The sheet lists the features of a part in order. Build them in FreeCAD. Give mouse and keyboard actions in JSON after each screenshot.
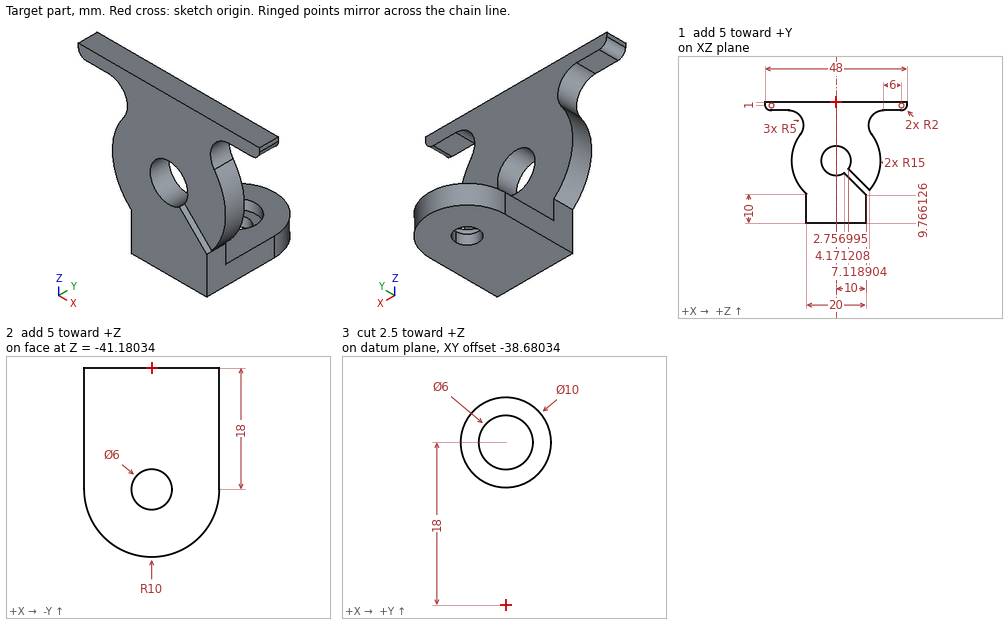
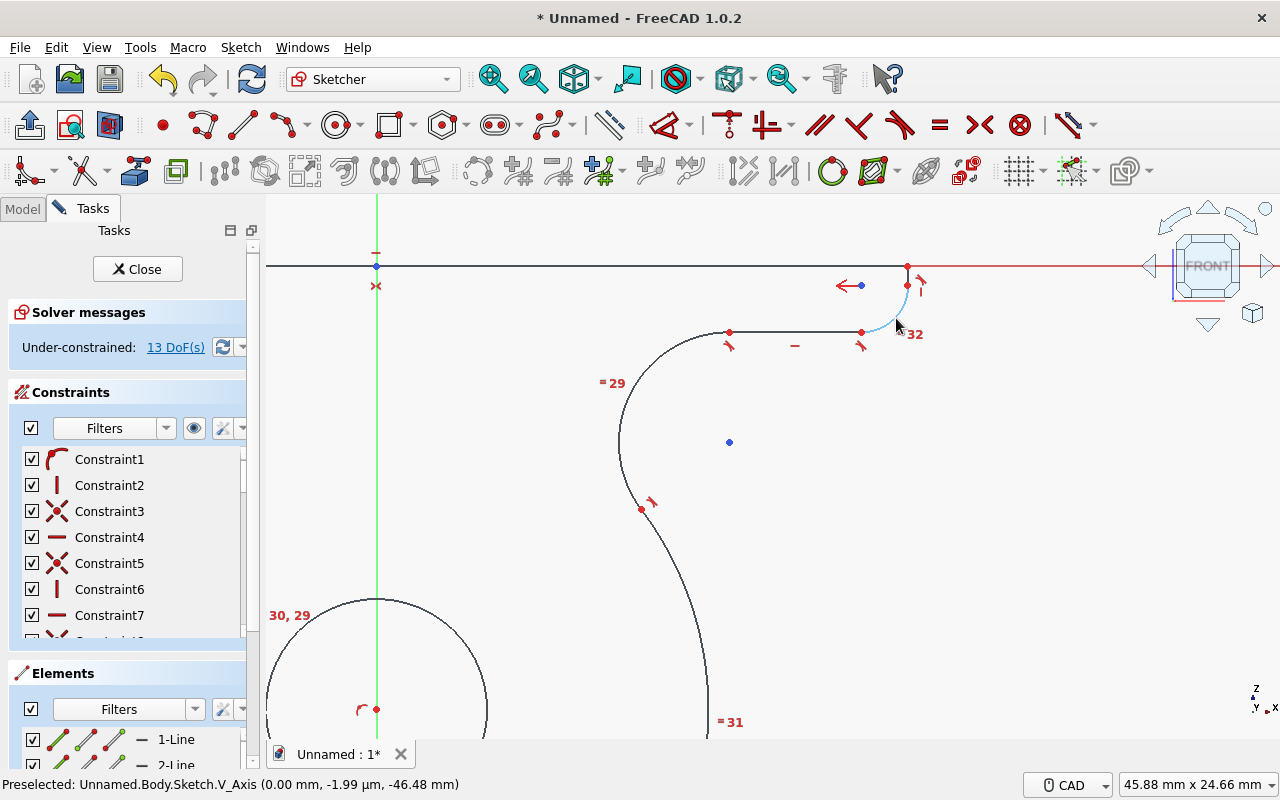
{"action": "left_click", "coordinate": [894, 319]}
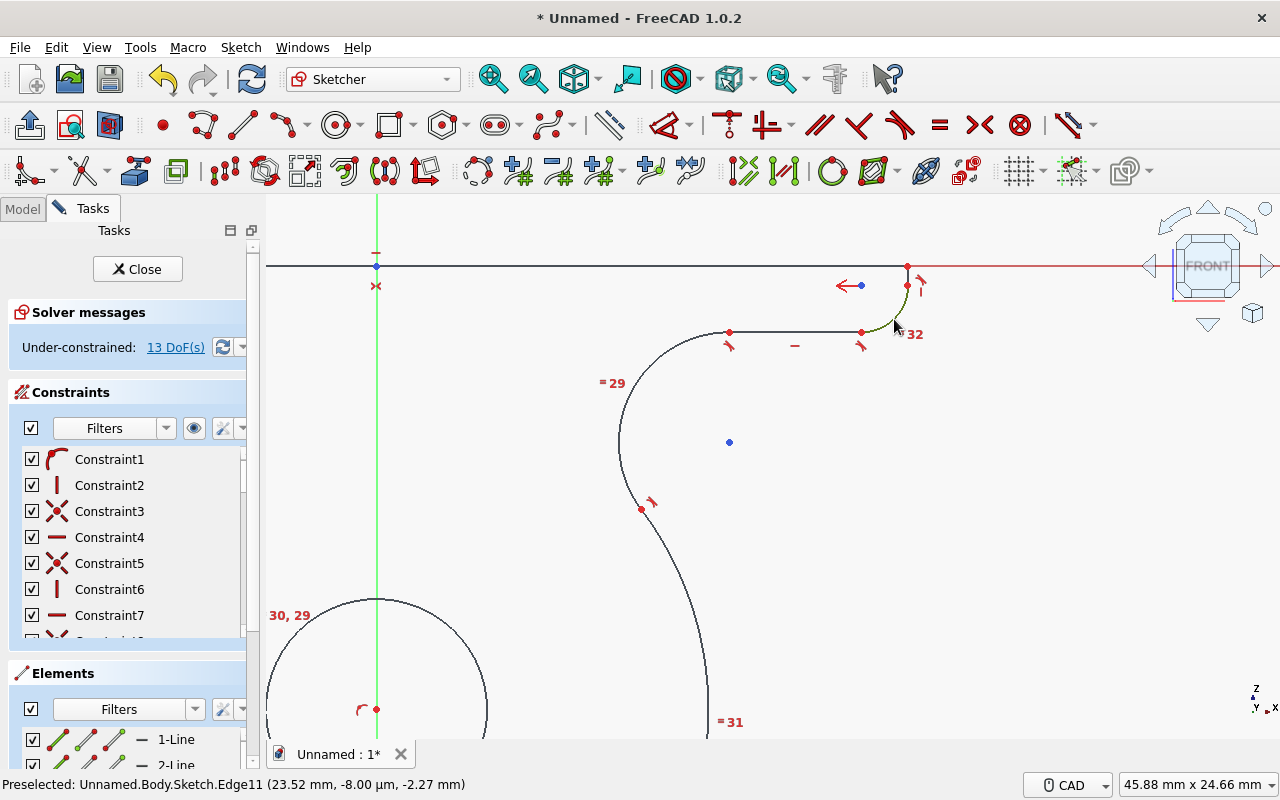
{"action": "key", "text": "k r"}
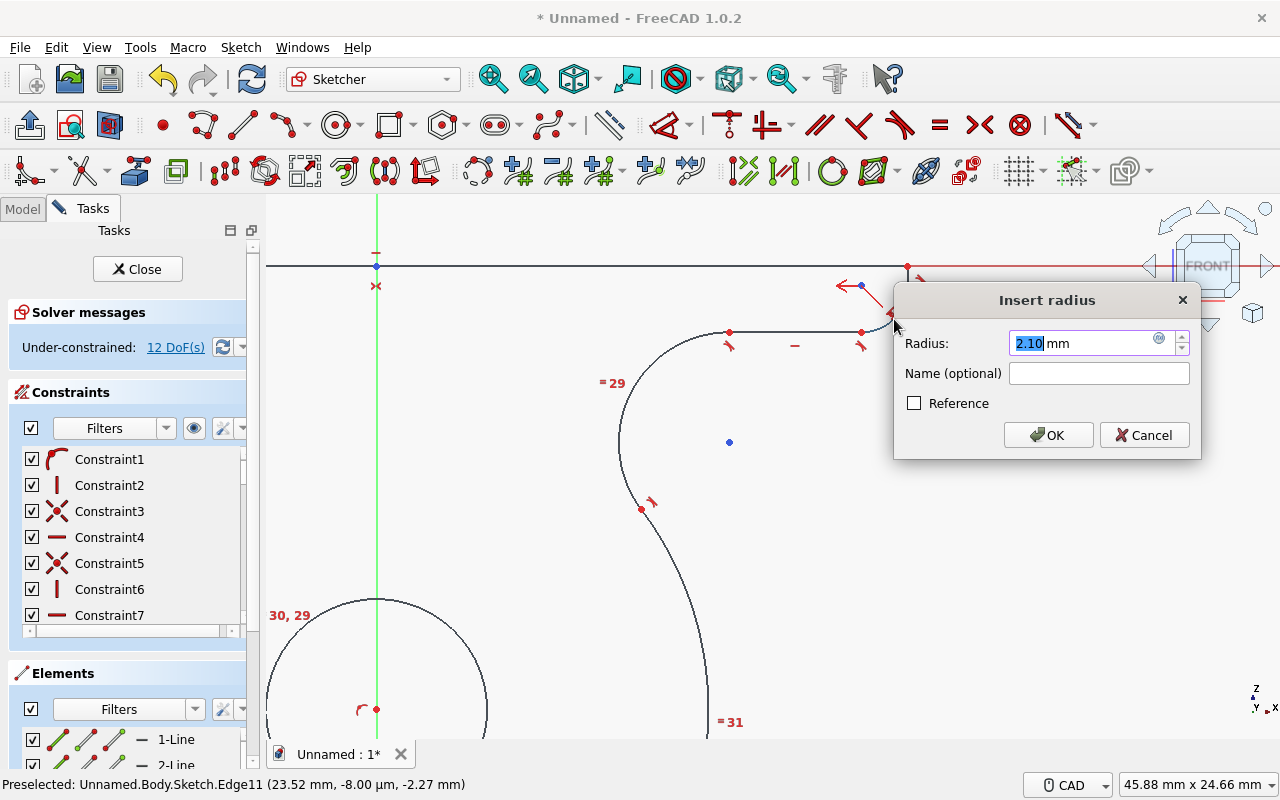
{"action": "type", "text": "2"}
{"action": "key", "text": "Return"}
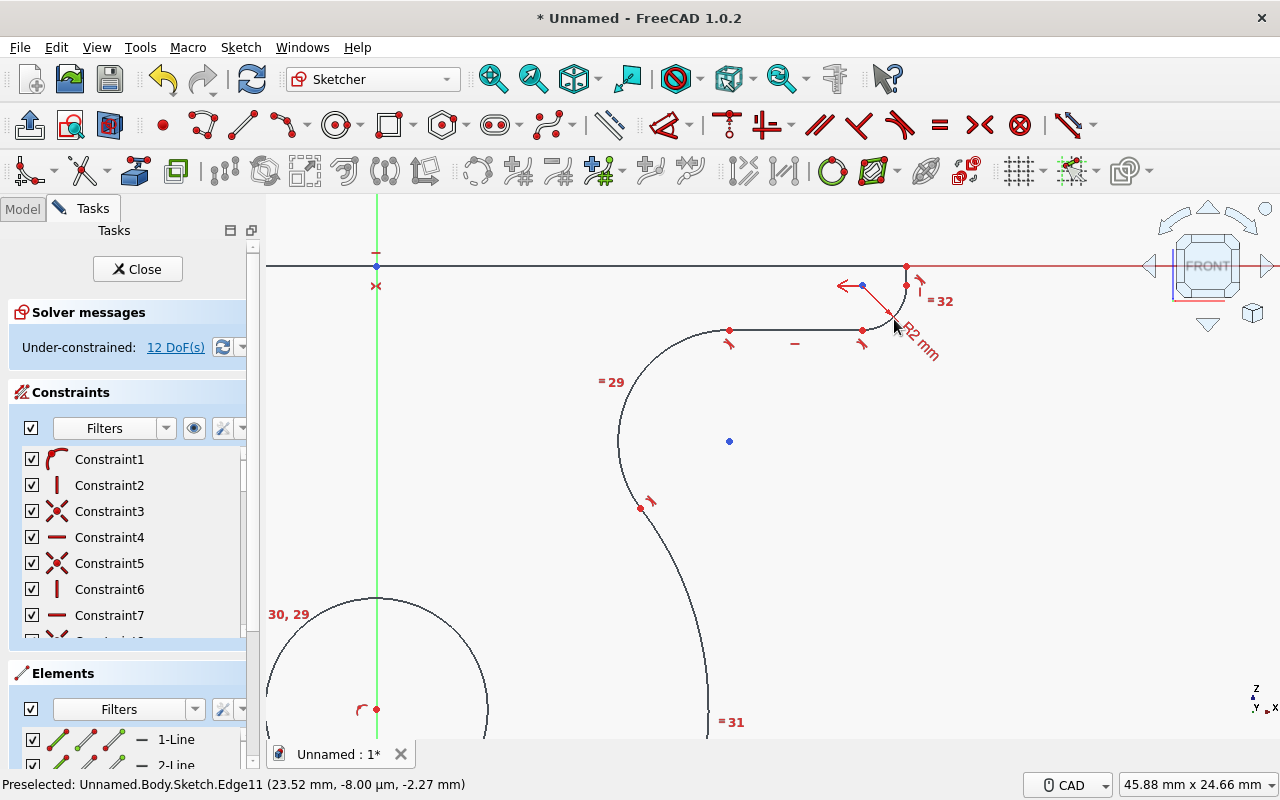
{"action": "left_click", "coordinate": [661, 354]}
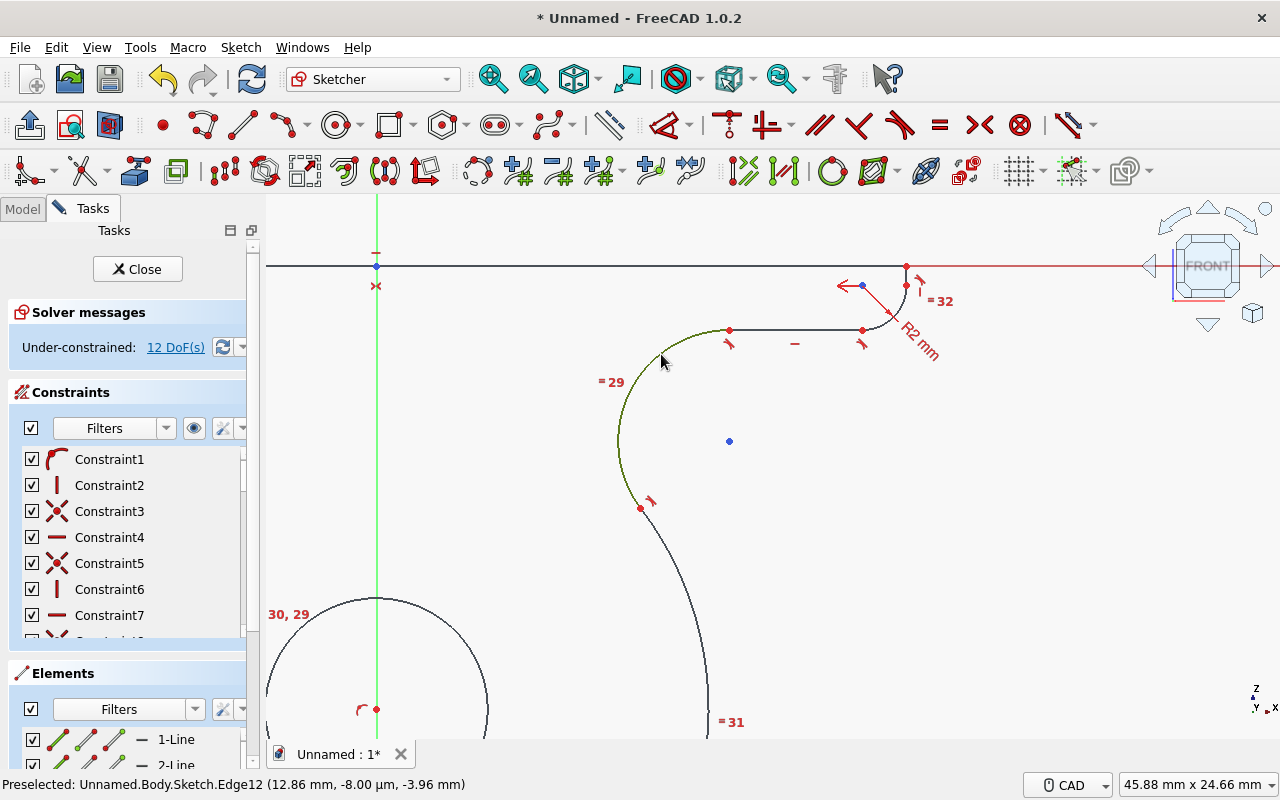
{"action": "key", "text": "k r"}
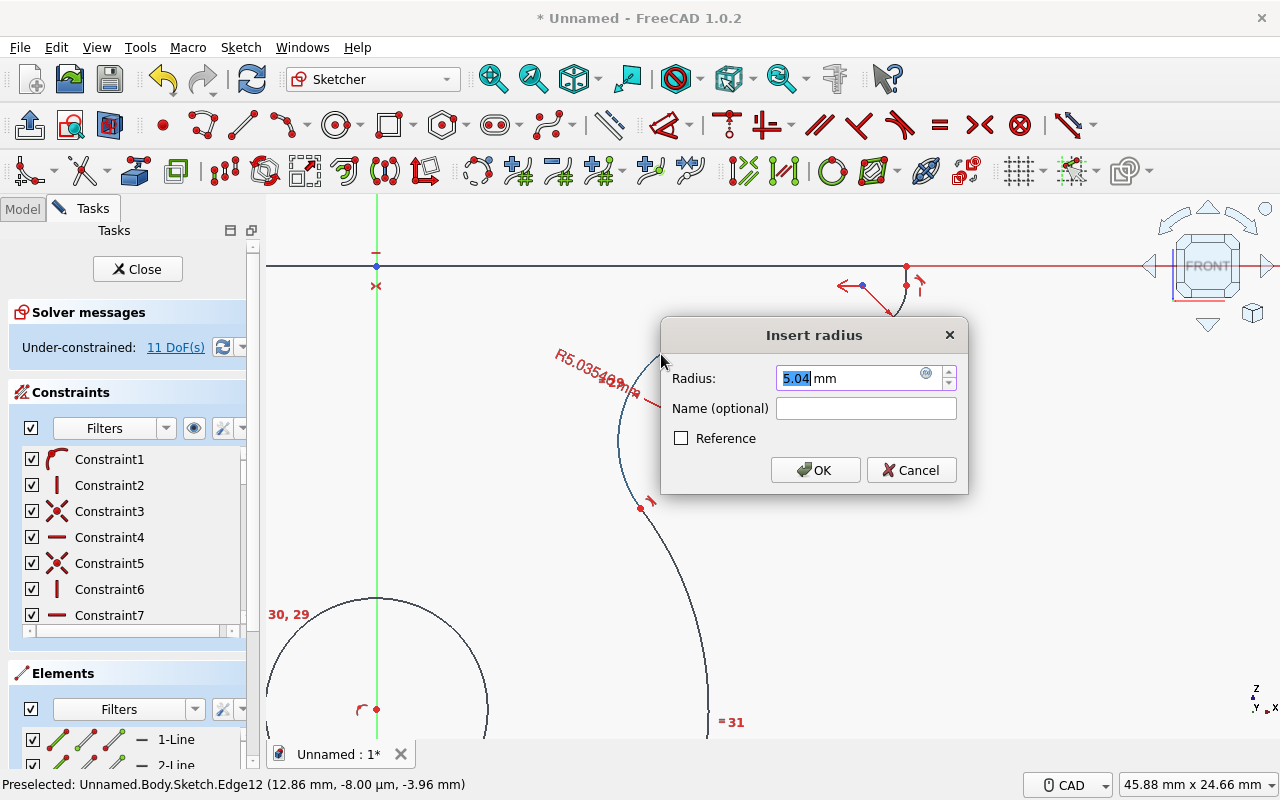
{"action": "type", "text": "5"}
{"action": "key", "text": "Return"}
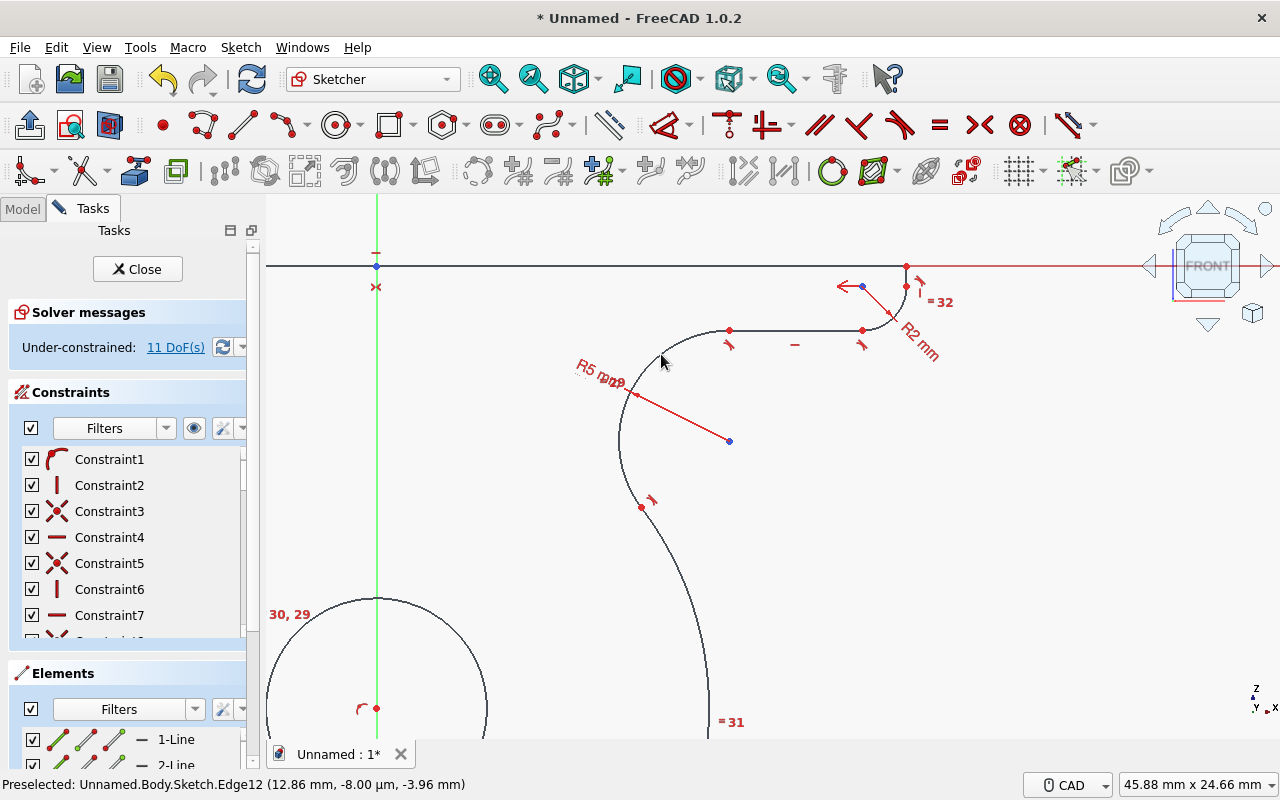
{"action": "left_click", "coordinate": [700, 631]}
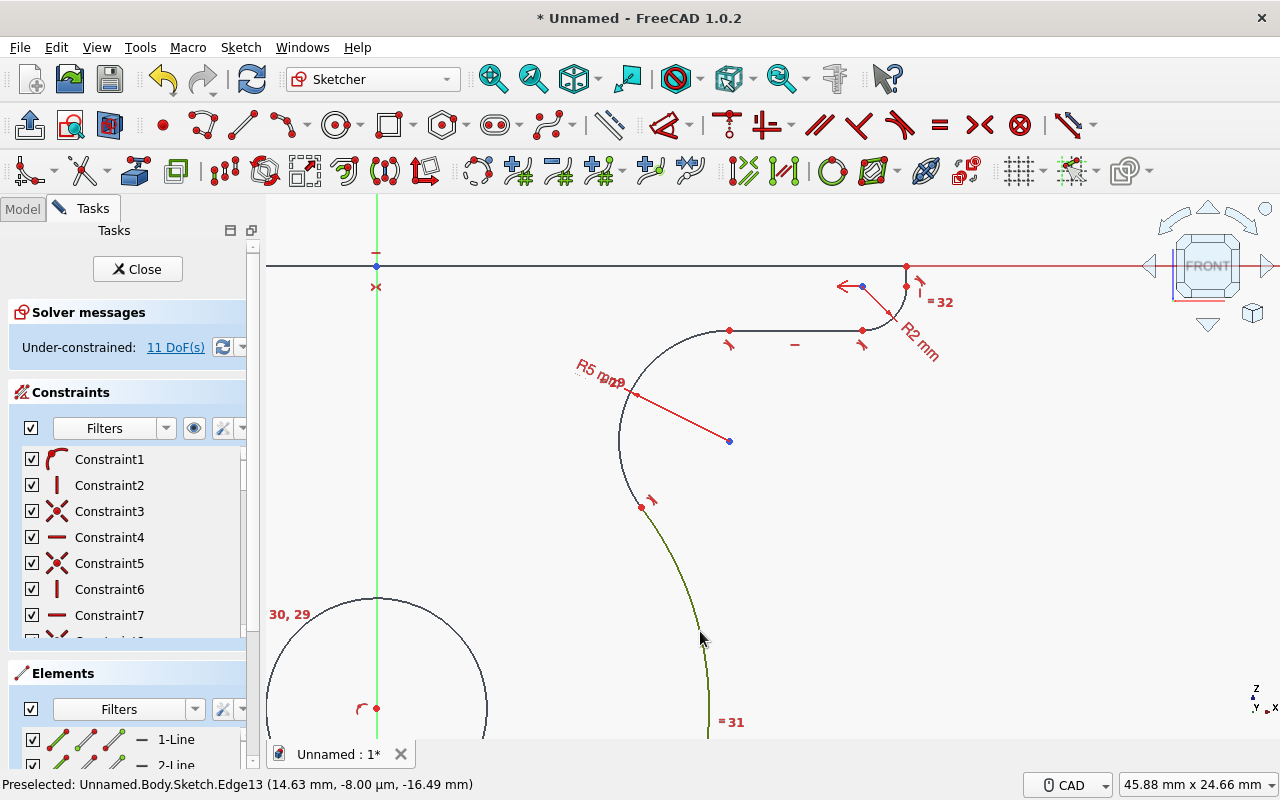
{"action": "key", "text": "k r"}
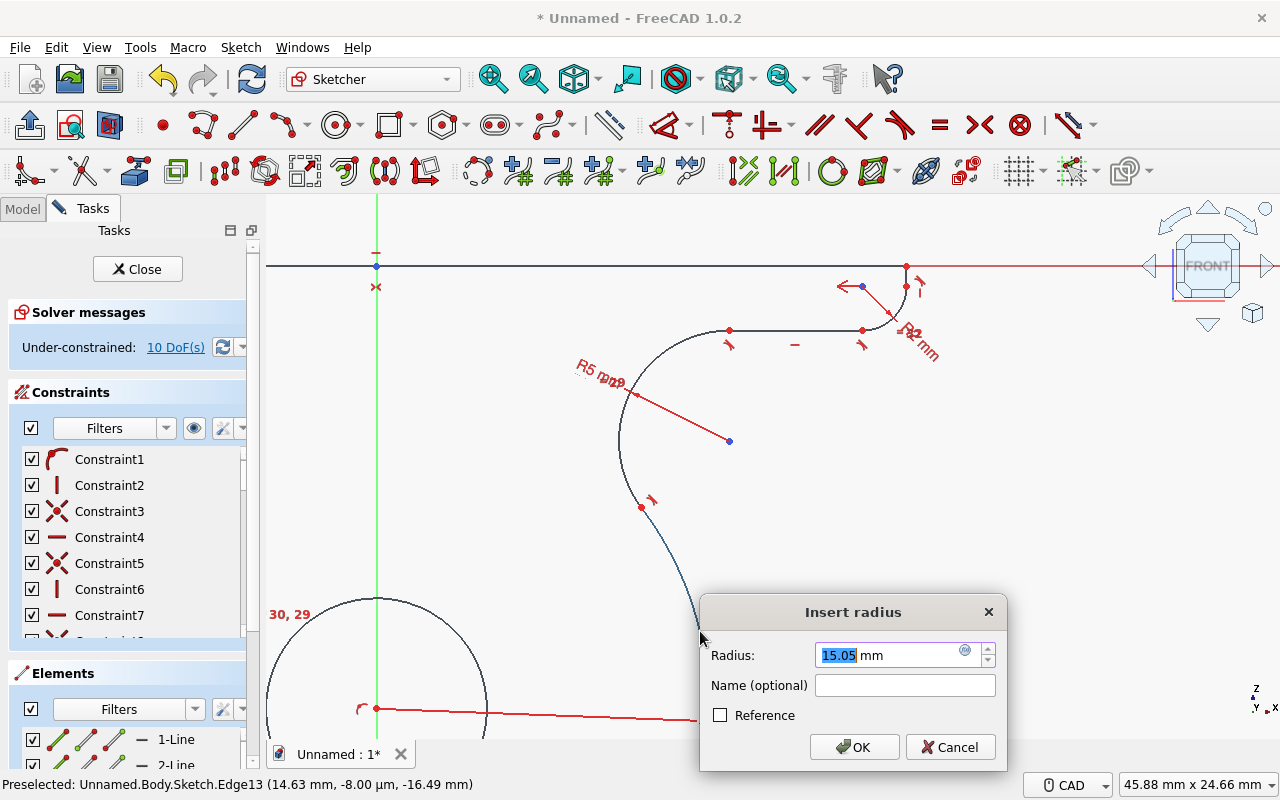
{"action": "type", "text": "15"}
{"action": "key", "text": "Return"}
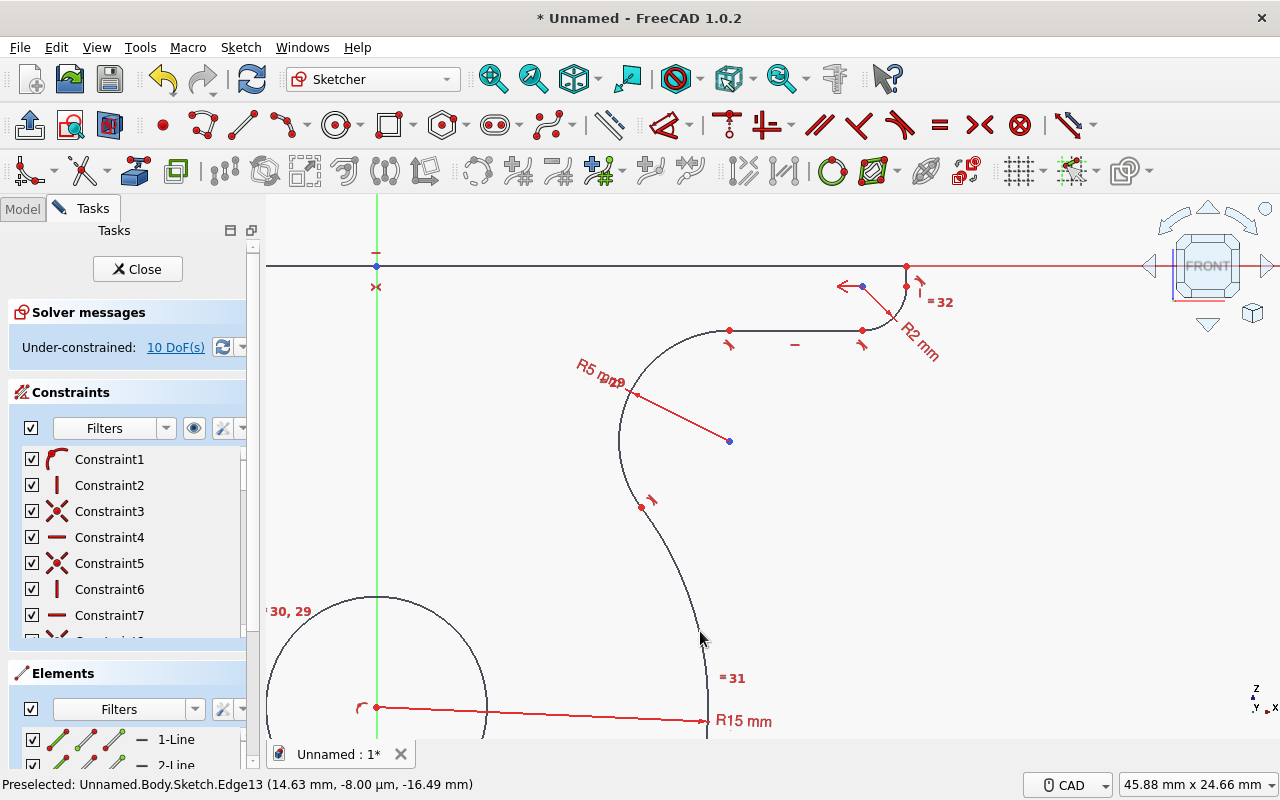
{"action": "scroll", "coordinate": [895, 318], "scroll_direction": "down", "scroll_amount": 5}